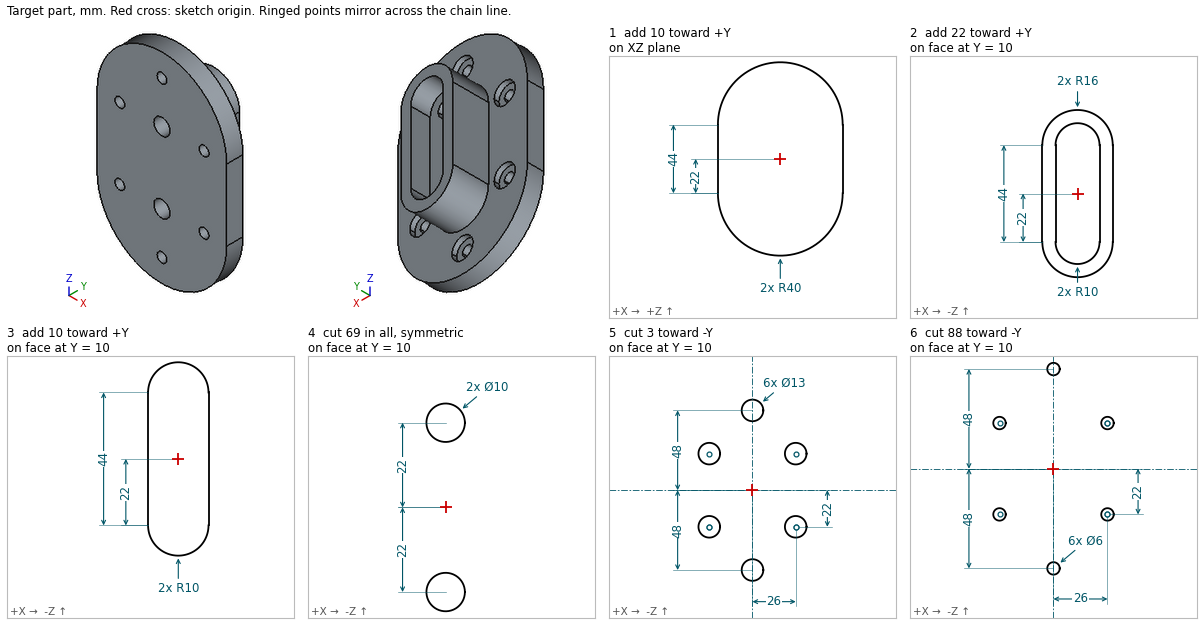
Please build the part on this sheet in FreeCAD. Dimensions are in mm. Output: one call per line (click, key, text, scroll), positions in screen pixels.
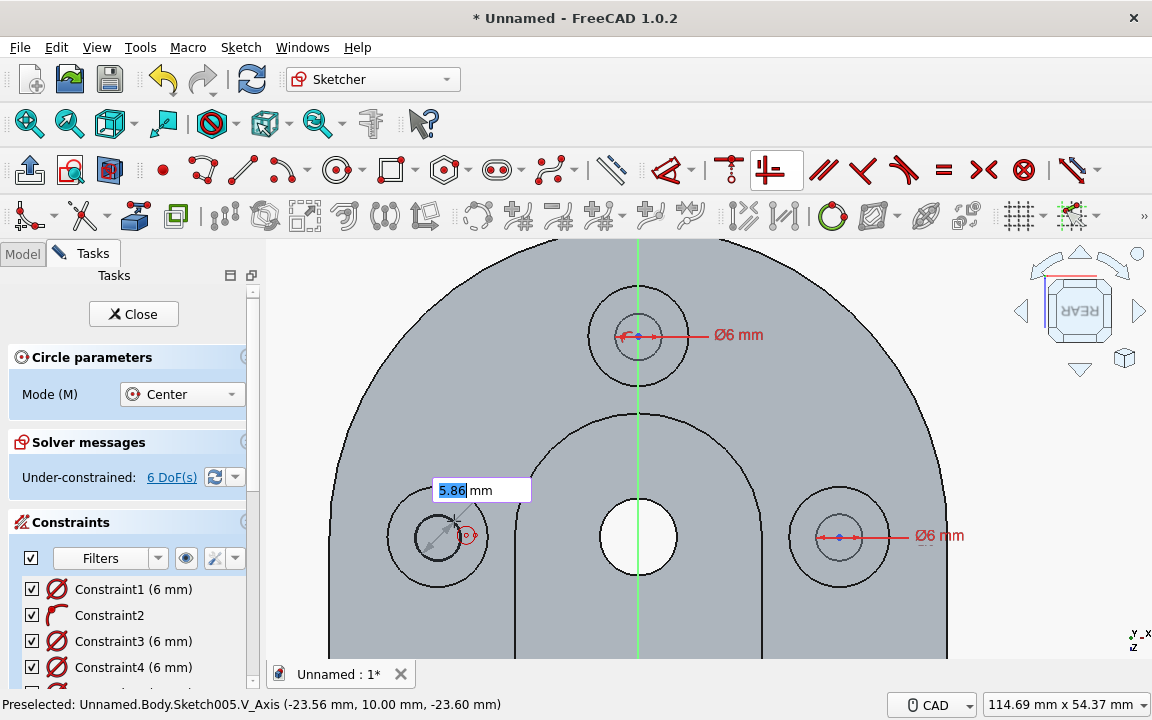
text(6)
key(Return)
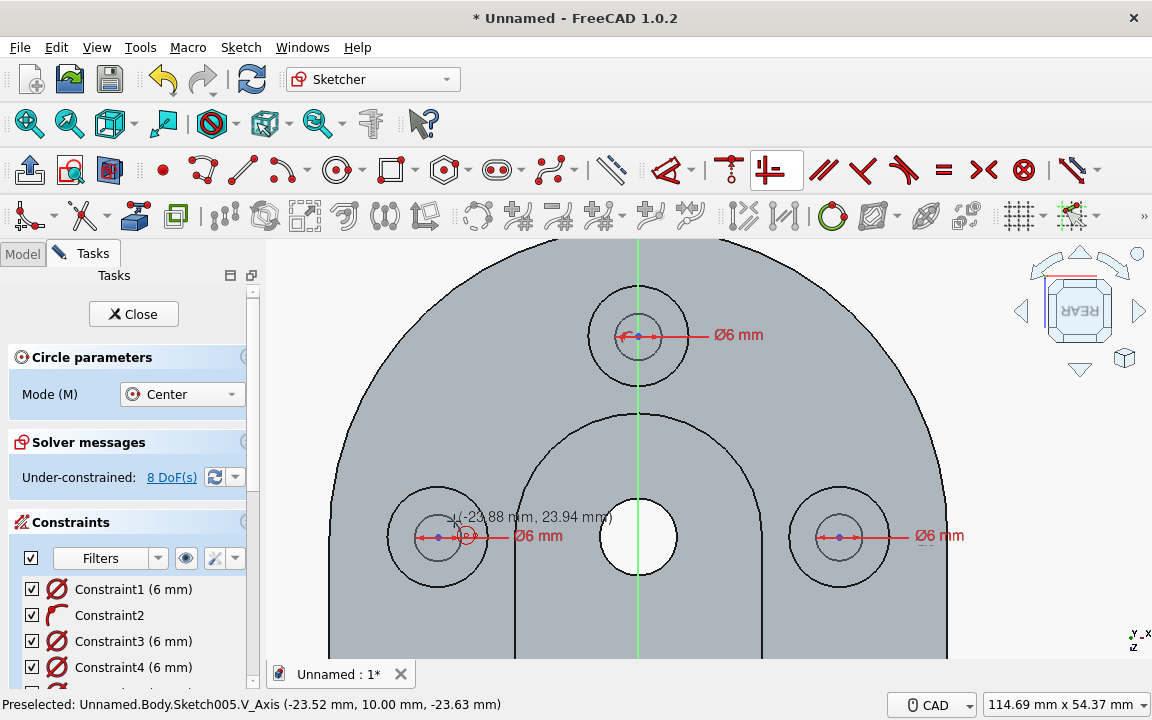
scroll(641, 338, down, 6)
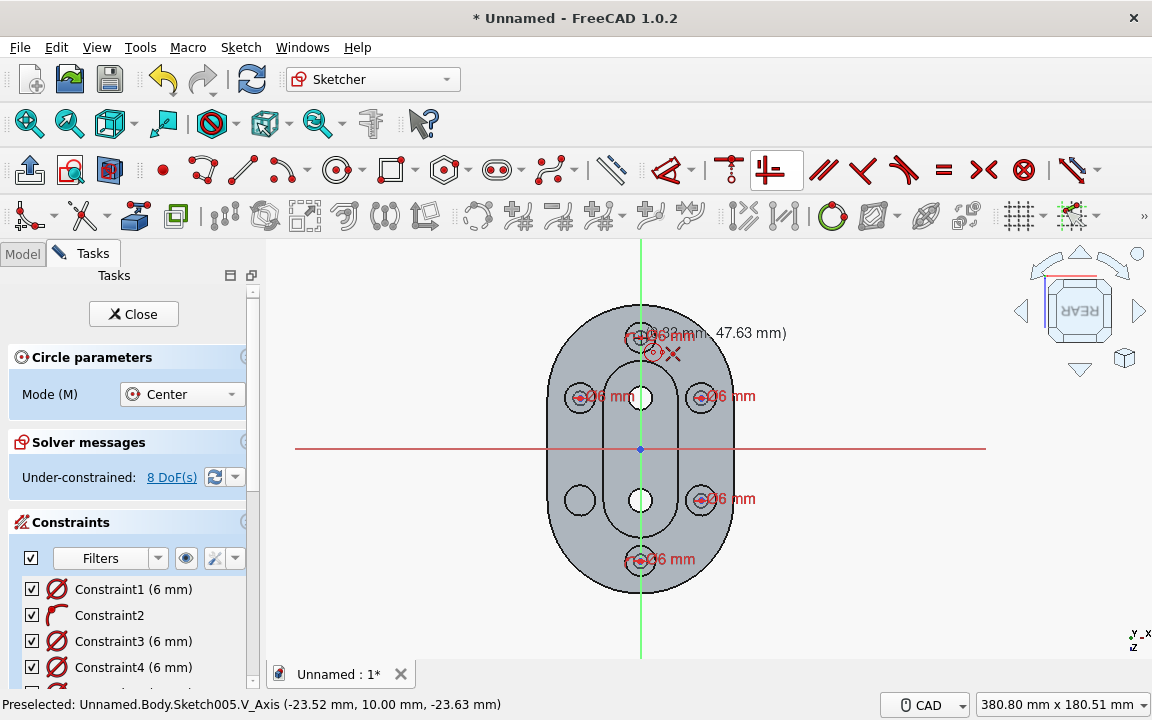
scroll(580, 500, up, 6)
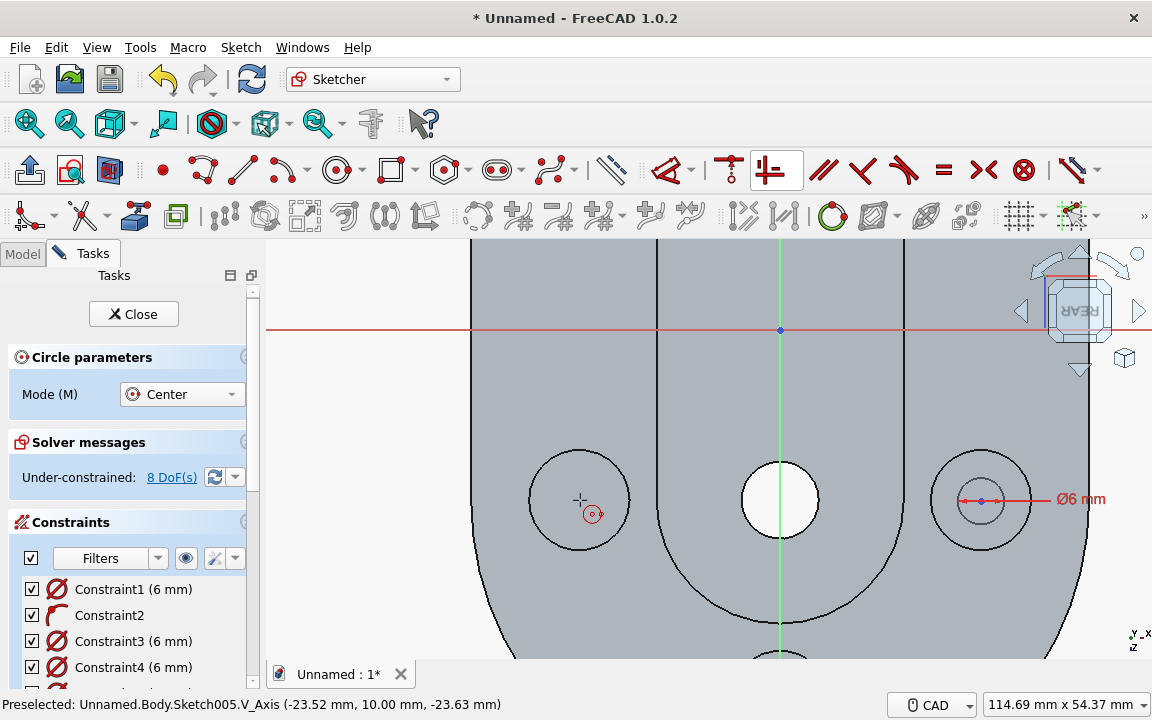
click(579, 500)
move(596, 484)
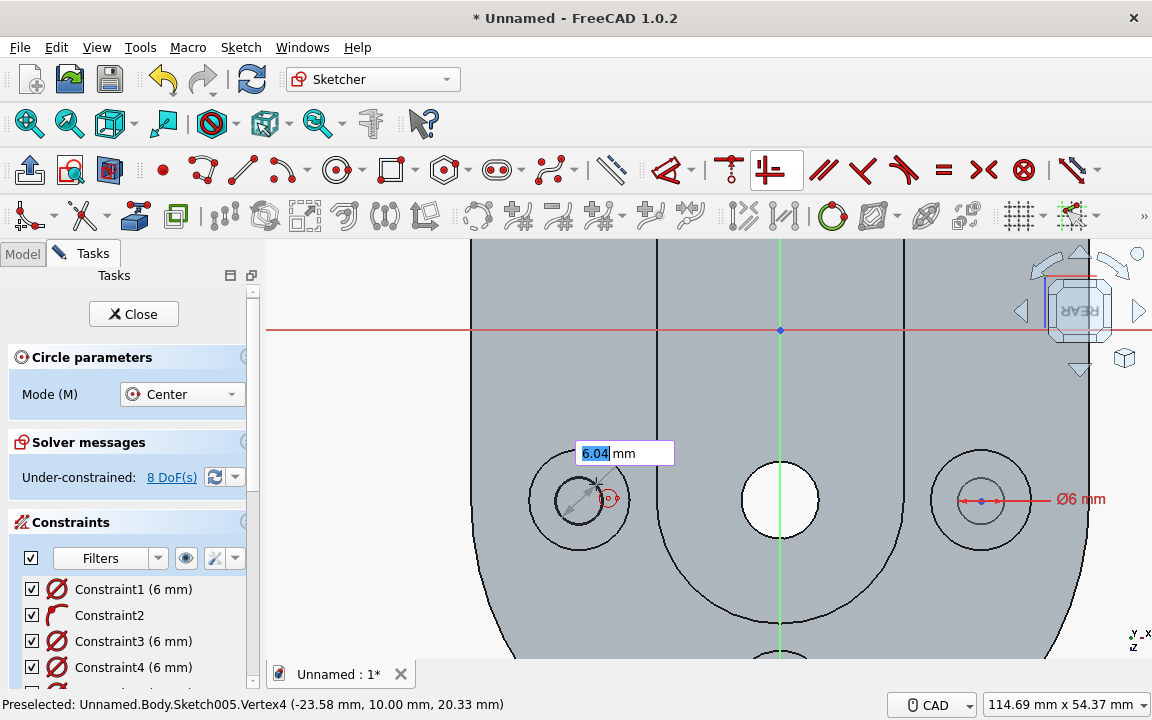
text(6)
key(Return)
key(Escape)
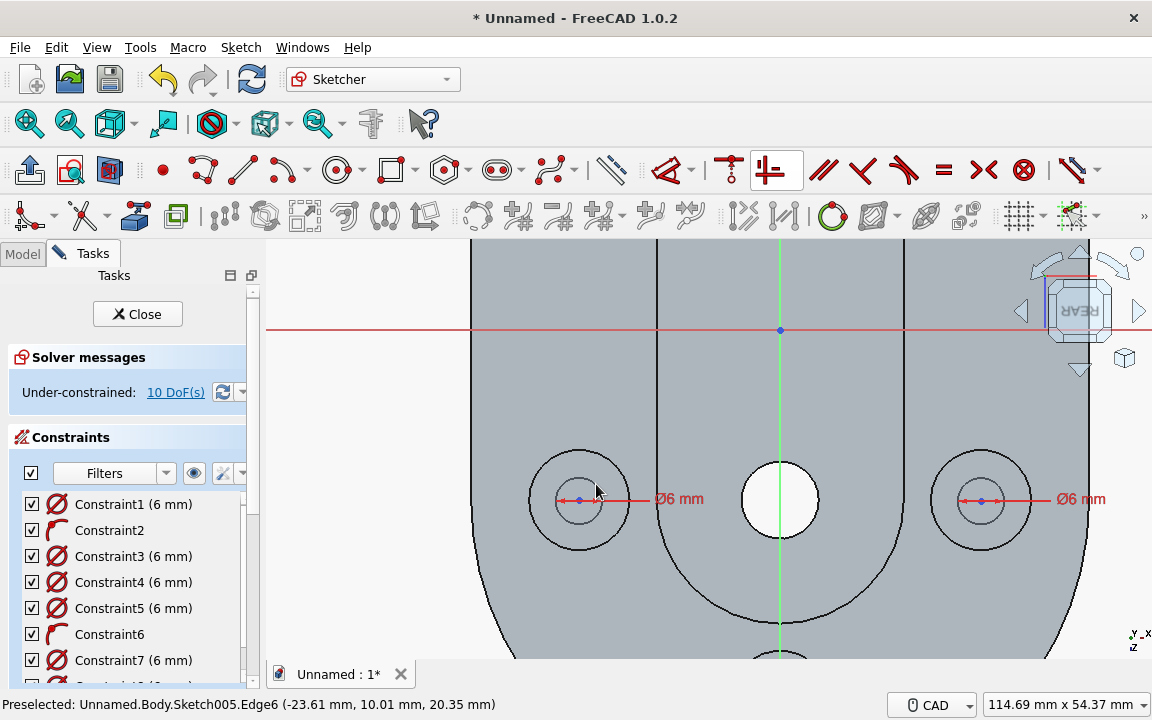
click(981, 501)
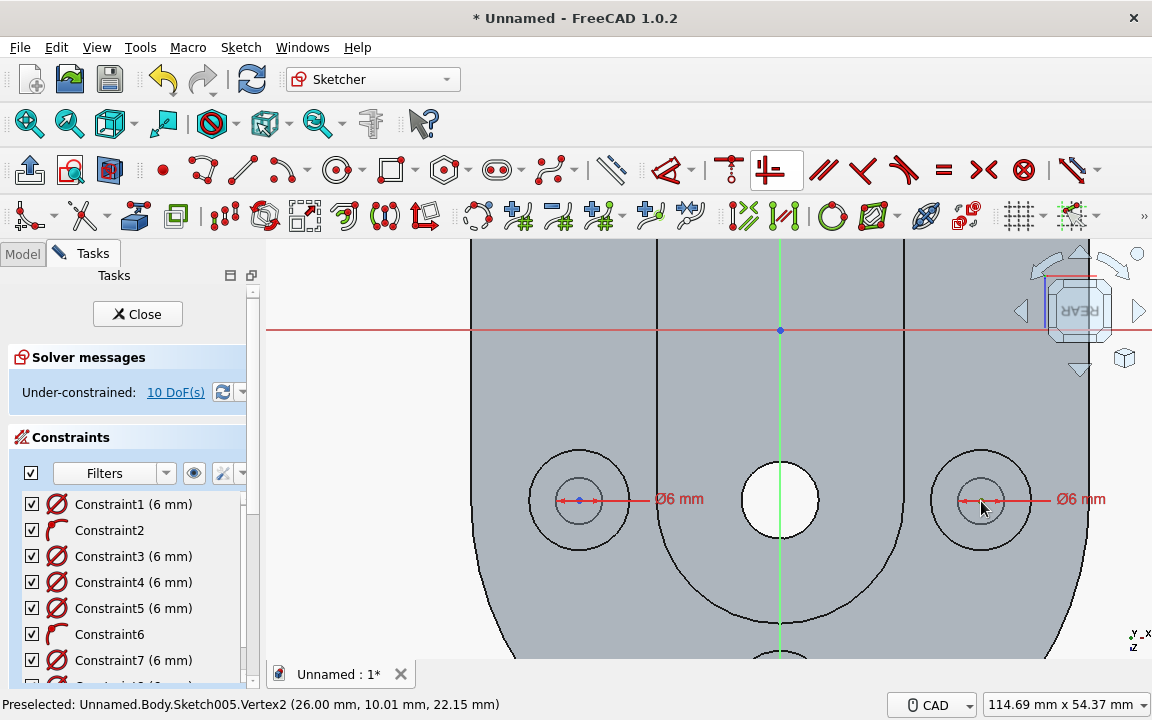
scroll(580, 500, down, 6)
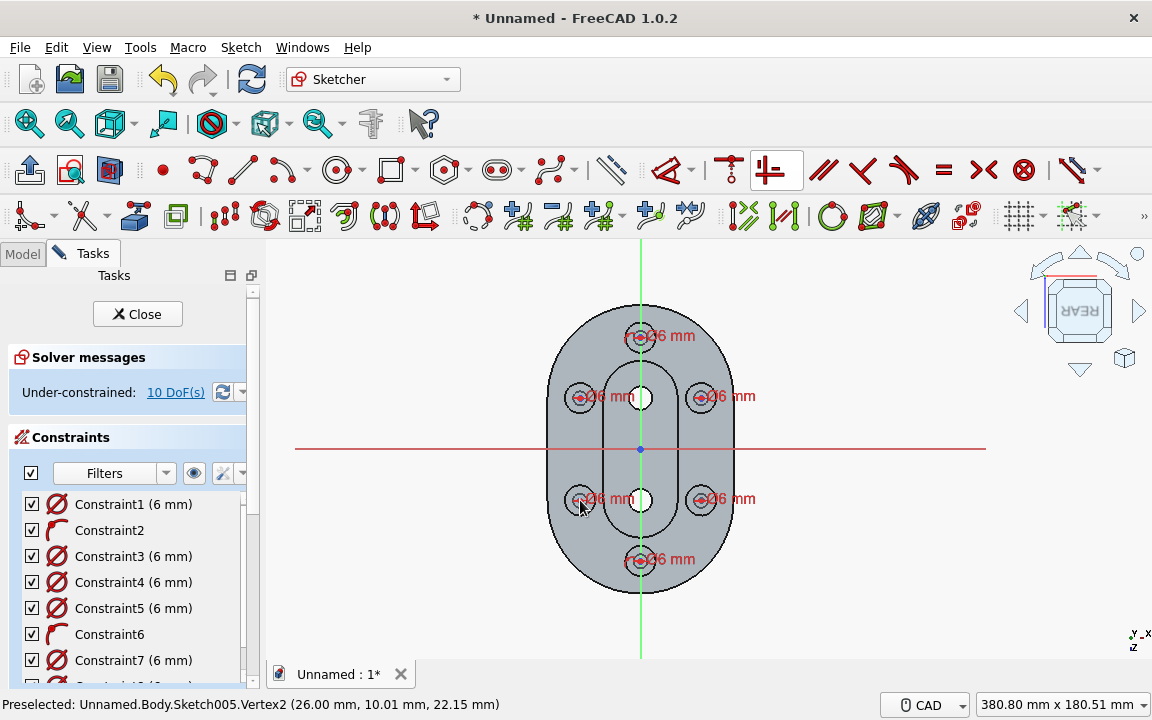
click(701, 398)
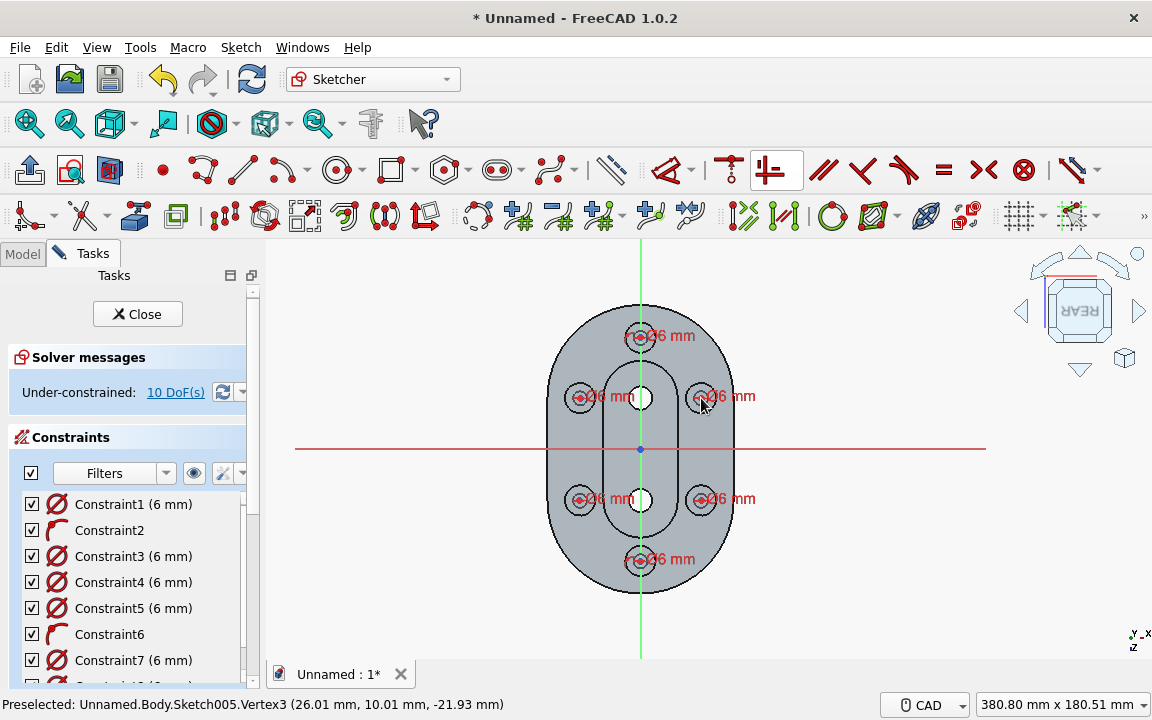
click(344, 449)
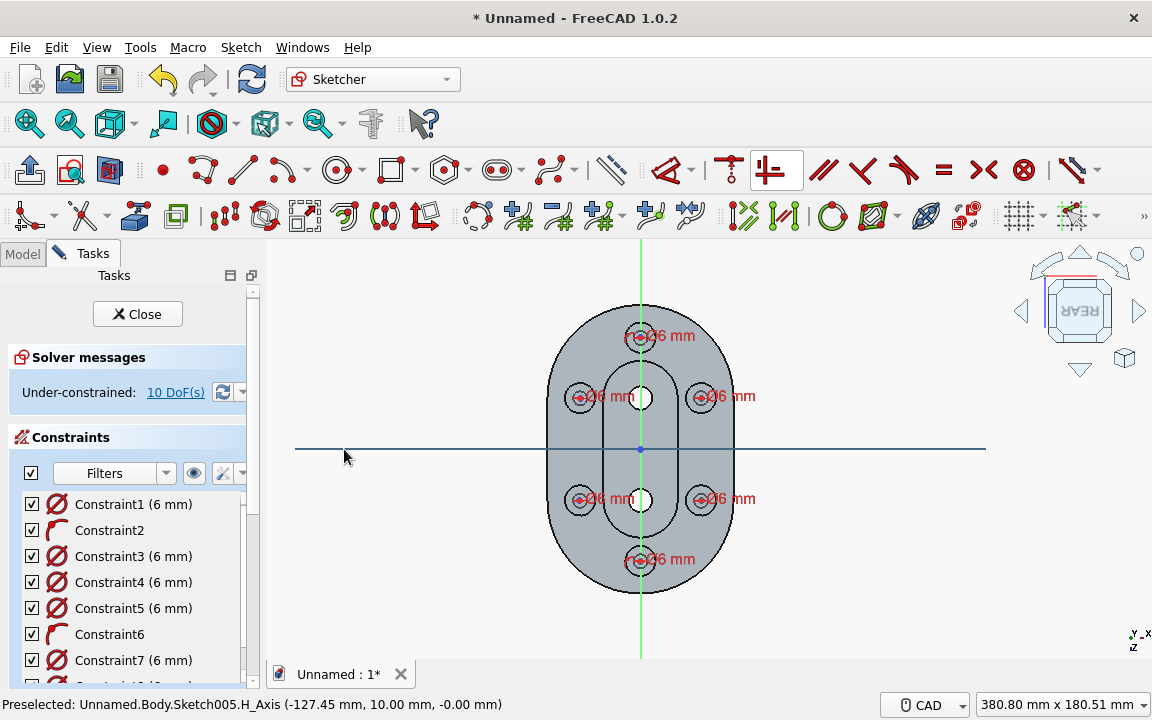
click(984, 170)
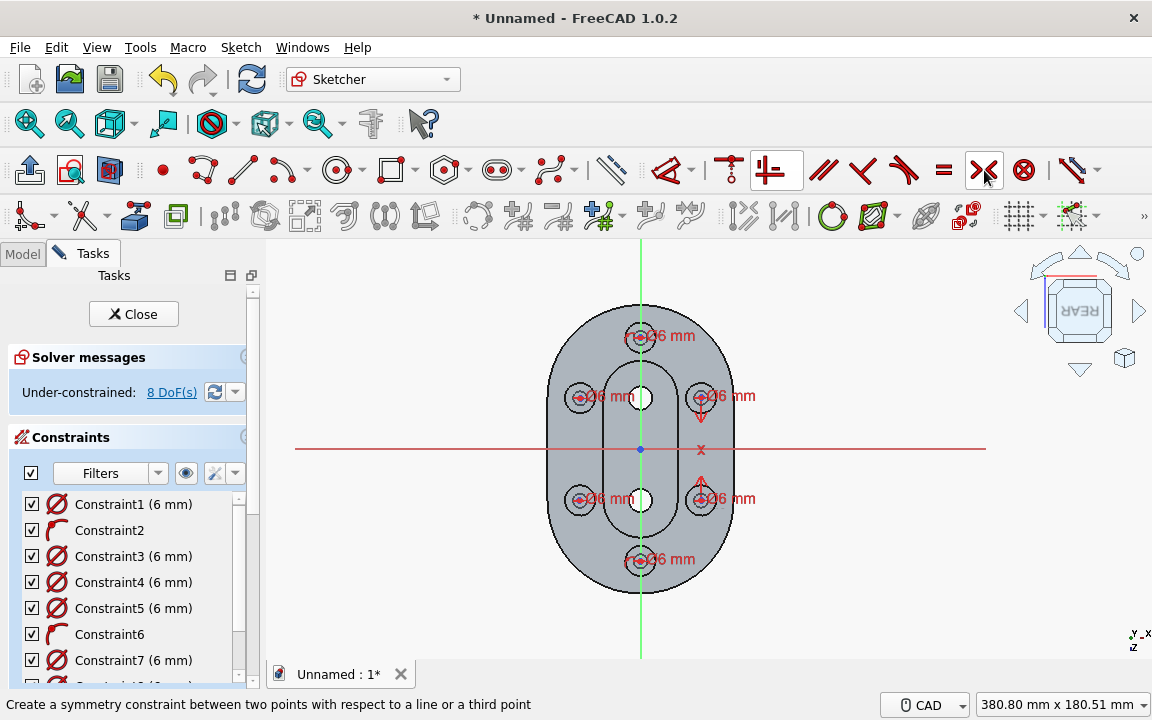
click(701, 398)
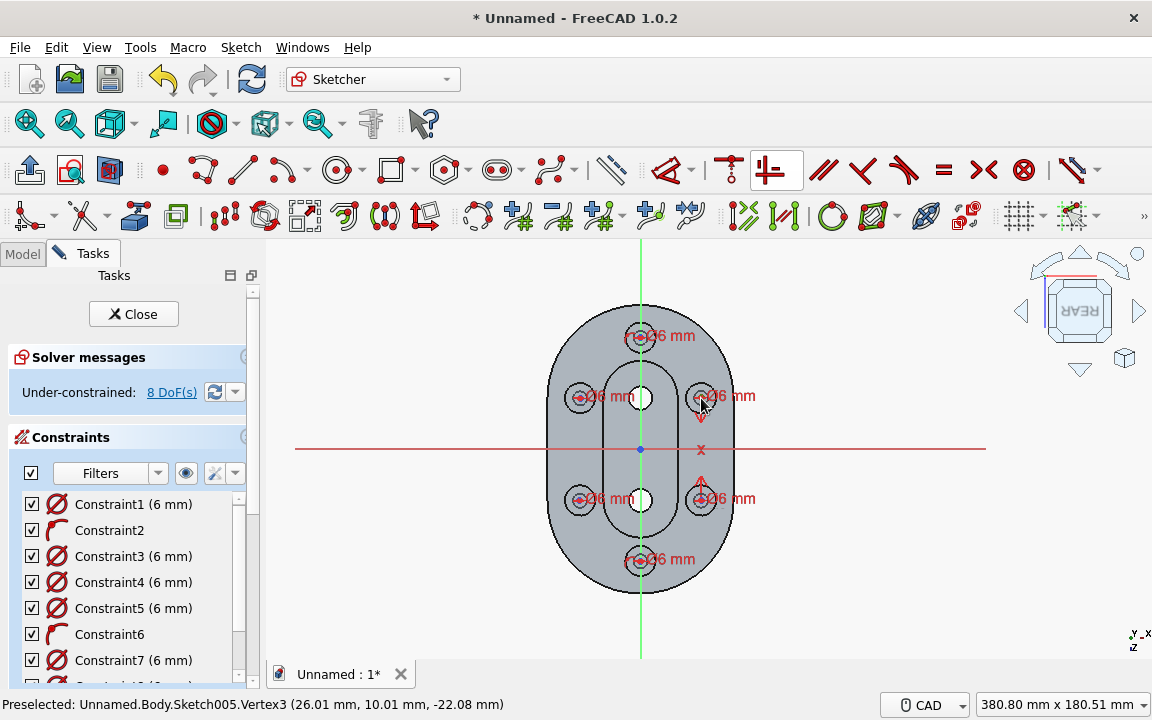
click(580, 398)